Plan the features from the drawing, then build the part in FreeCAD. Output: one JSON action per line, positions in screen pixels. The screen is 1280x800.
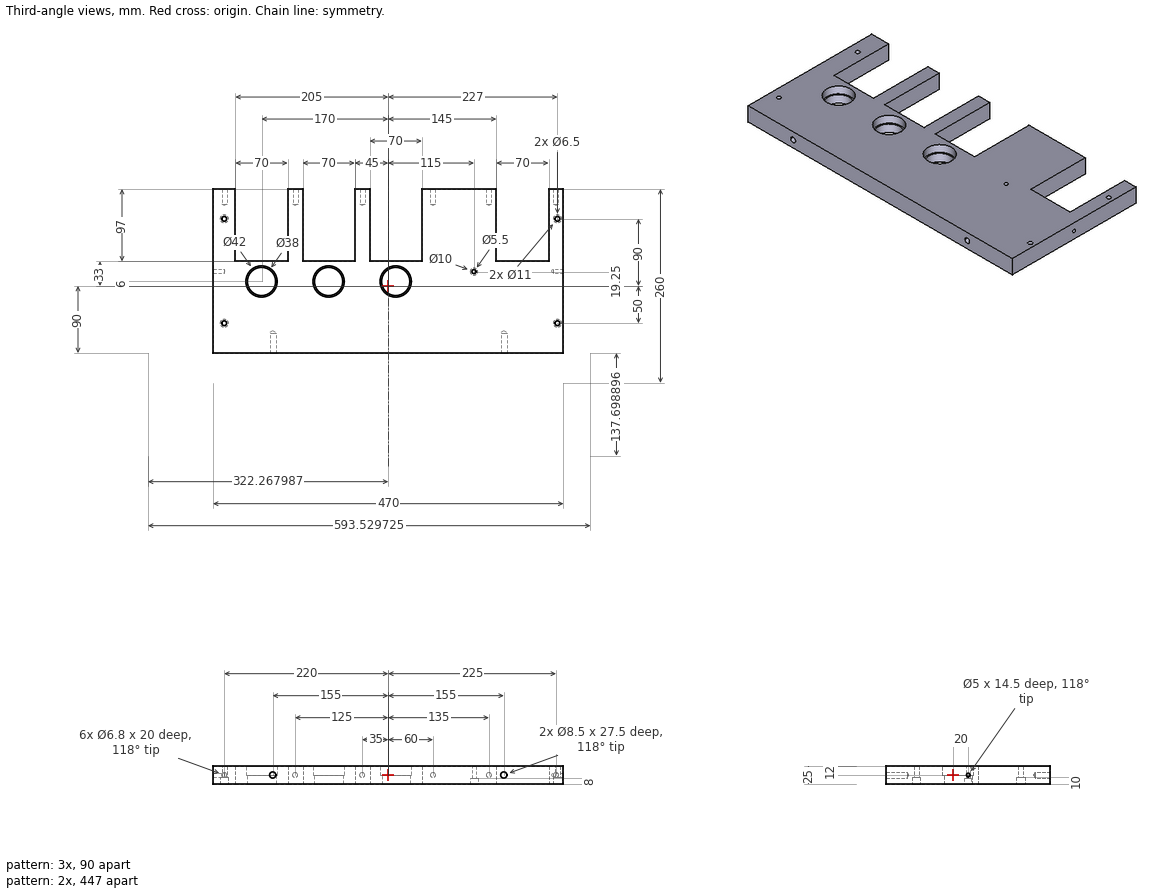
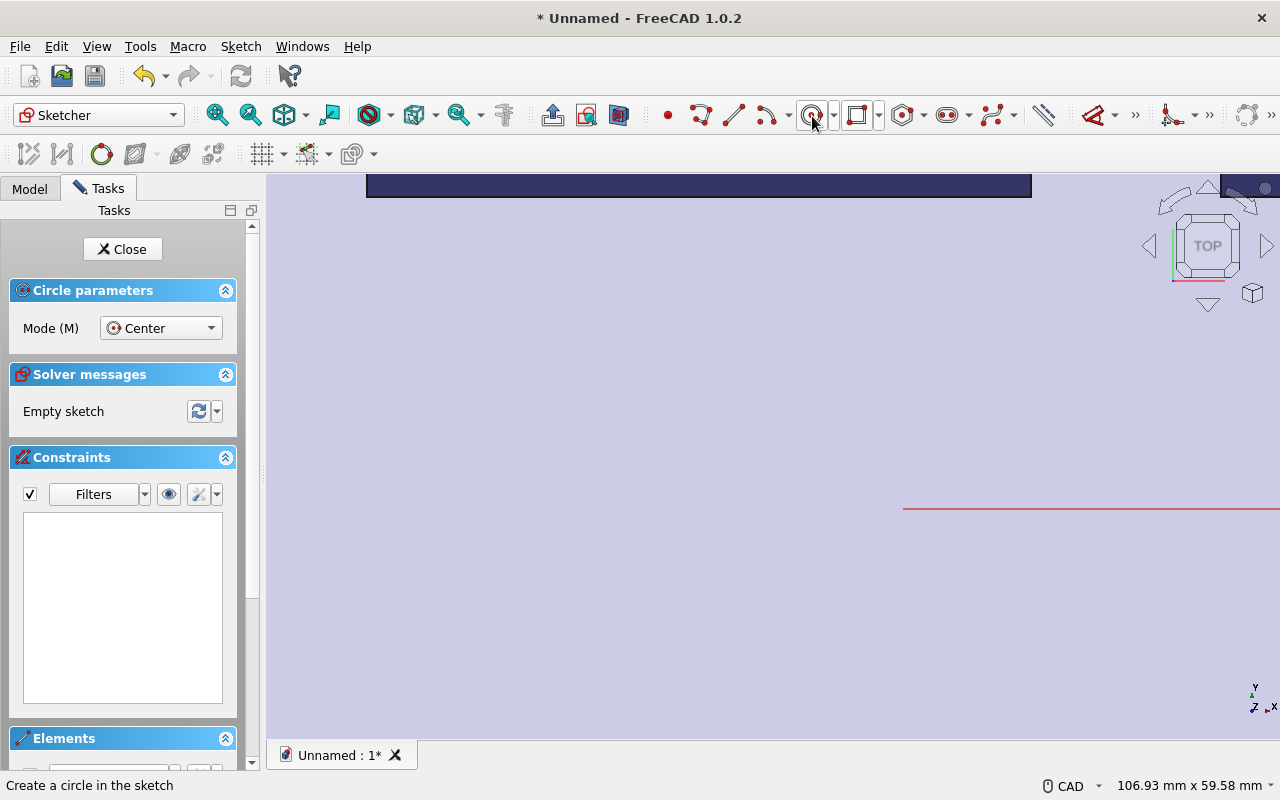
{"action": "left_click", "coordinate": [699, 453]}
{"action": "mouse_move", "coordinate": [827, 325]}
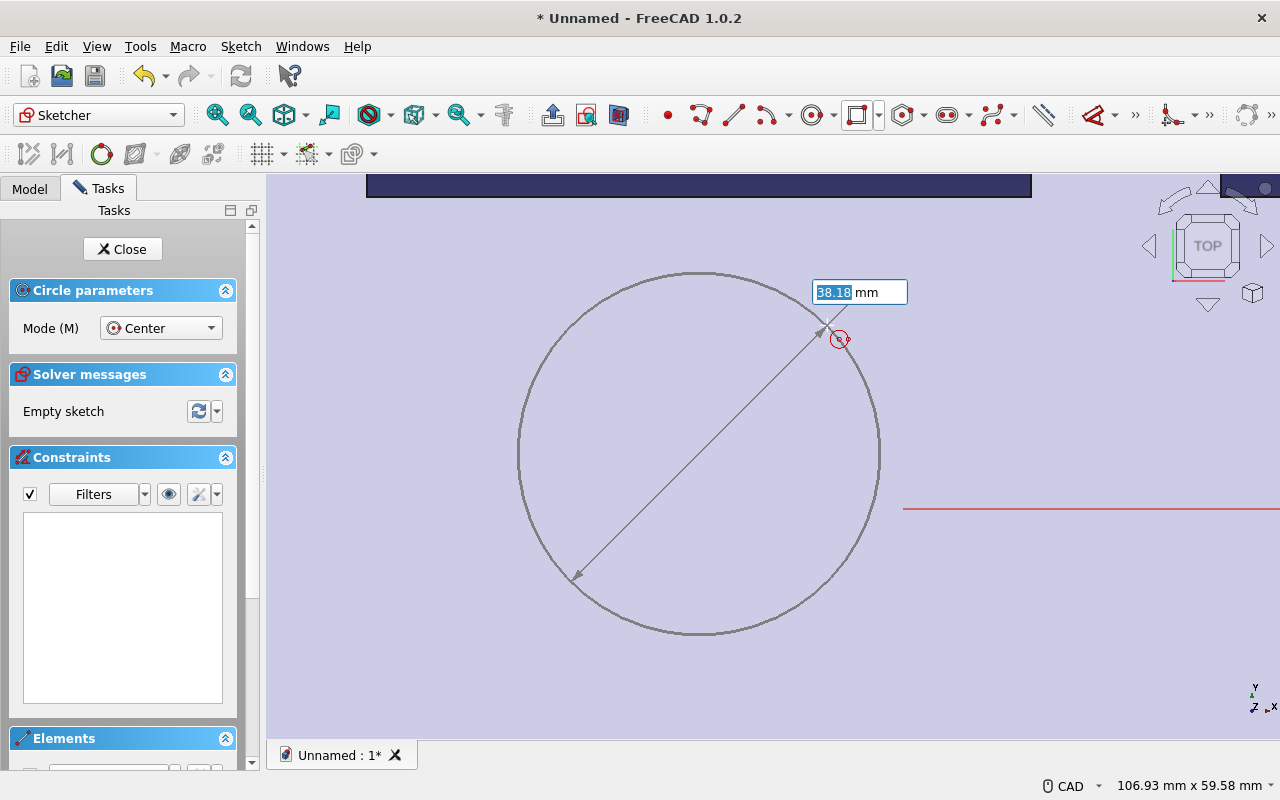
{"action": "type", "text": "38"}
{"action": "key", "text": "Return"}
{"action": "key", "text": "Escape"}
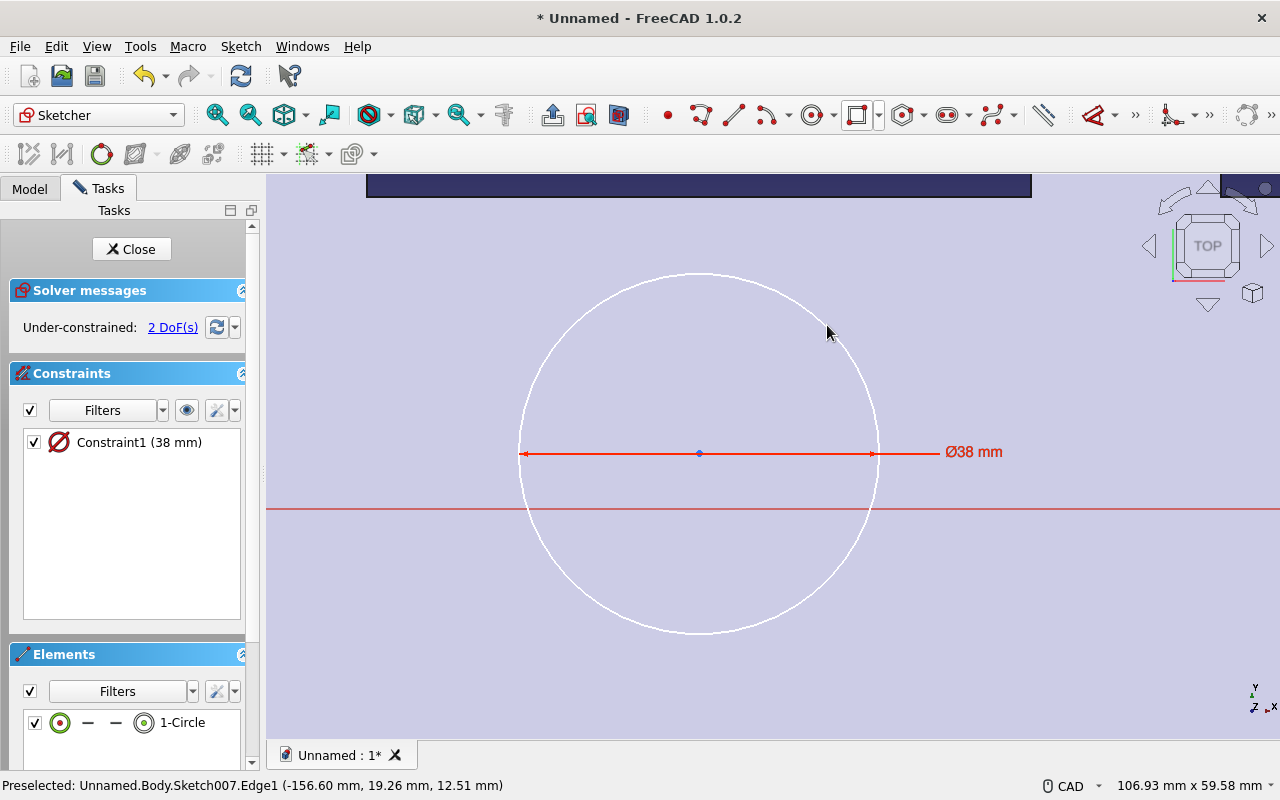
{"action": "left_click", "coordinate": [1092, 116]}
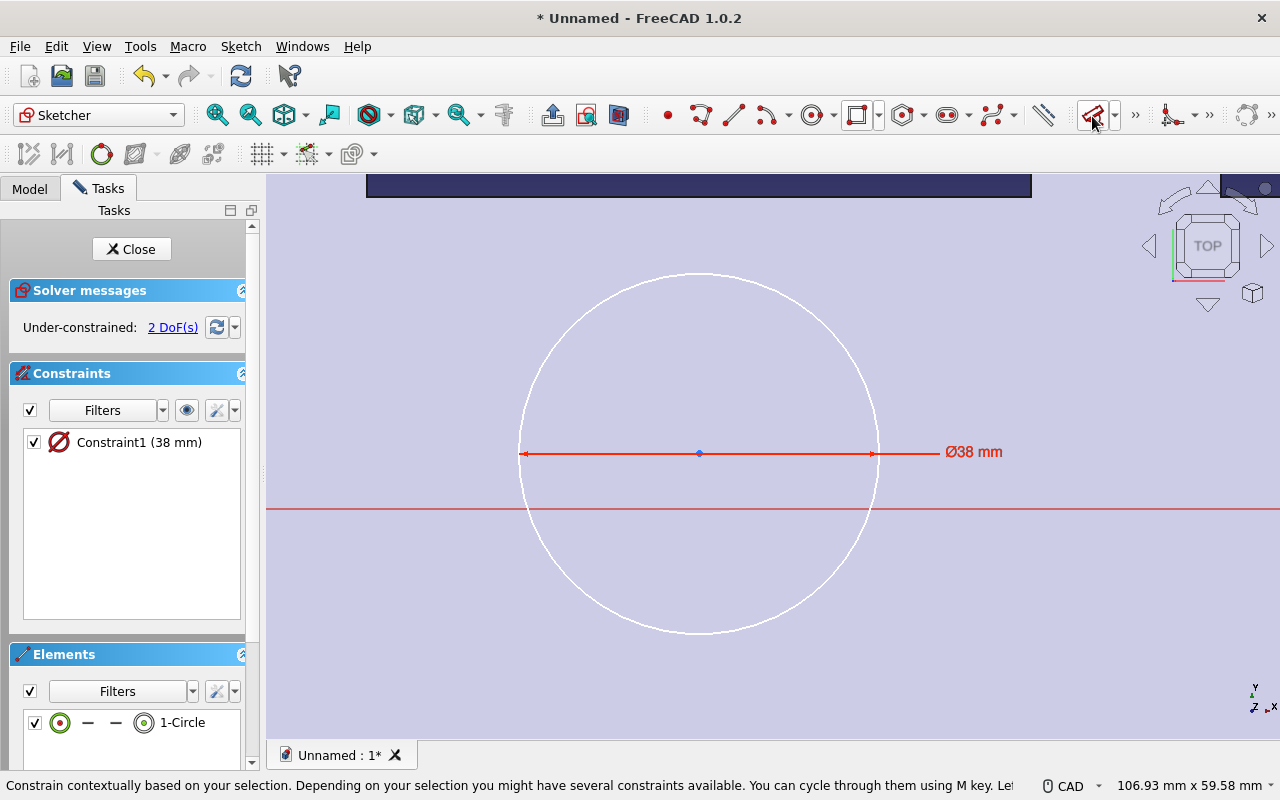
{"action": "left_click", "coordinate": [699, 454]}
{"action": "left_click", "coordinate": [665, 482]}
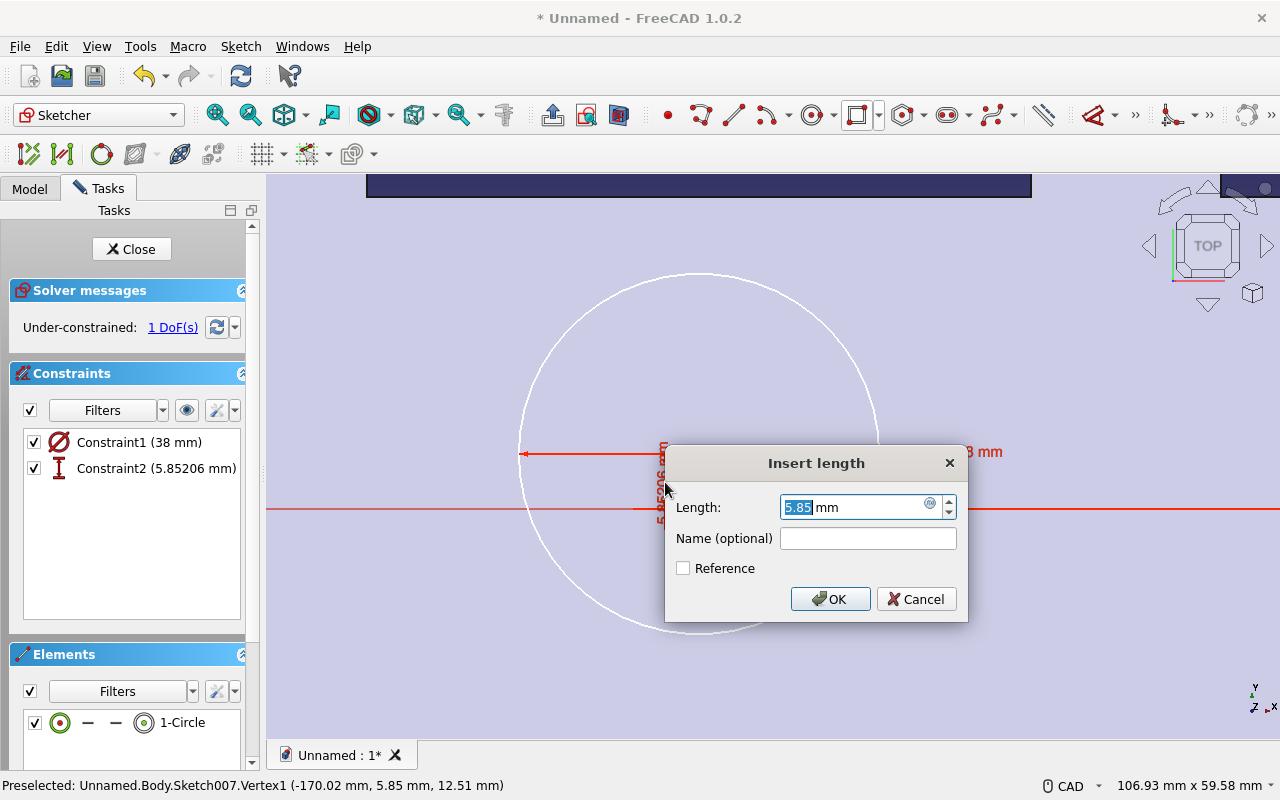
{"action": "type", "text": "6"}
{"action": "key", "text": "Return"}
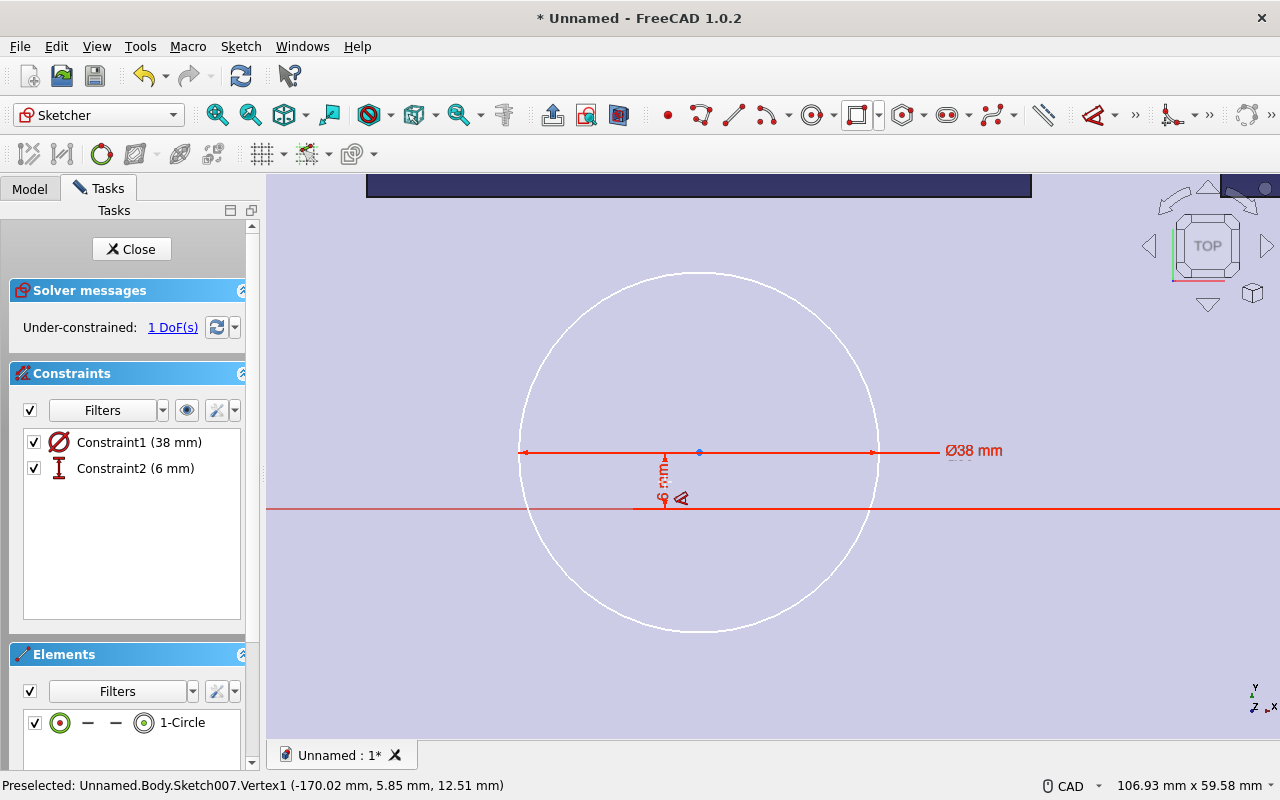
{"action": "left_click", "coordinate": [699, 453]}
{"action": "left_click", "coordinate": [907, 543]}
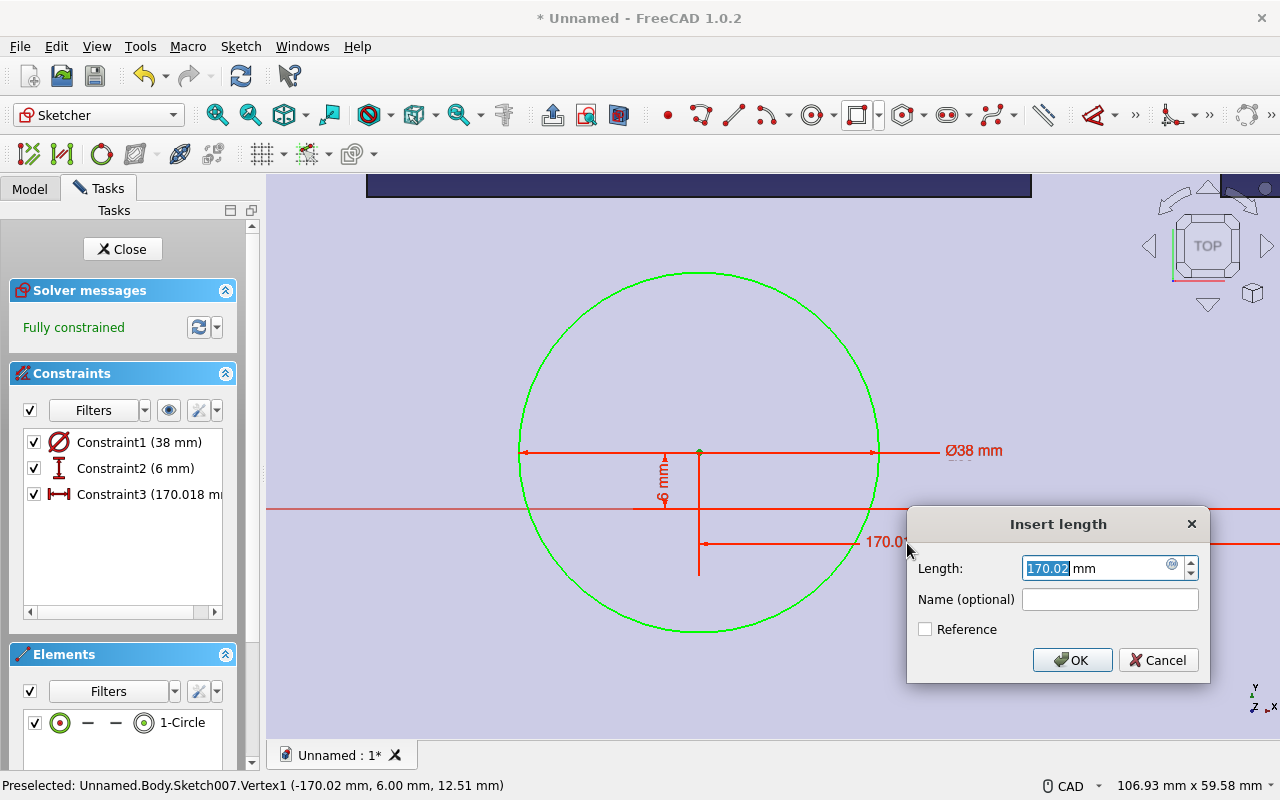
{"action": "type", "text": "170"}
{"action": "key", "text": "Return"}
{"action": "key", "text": "Escape"}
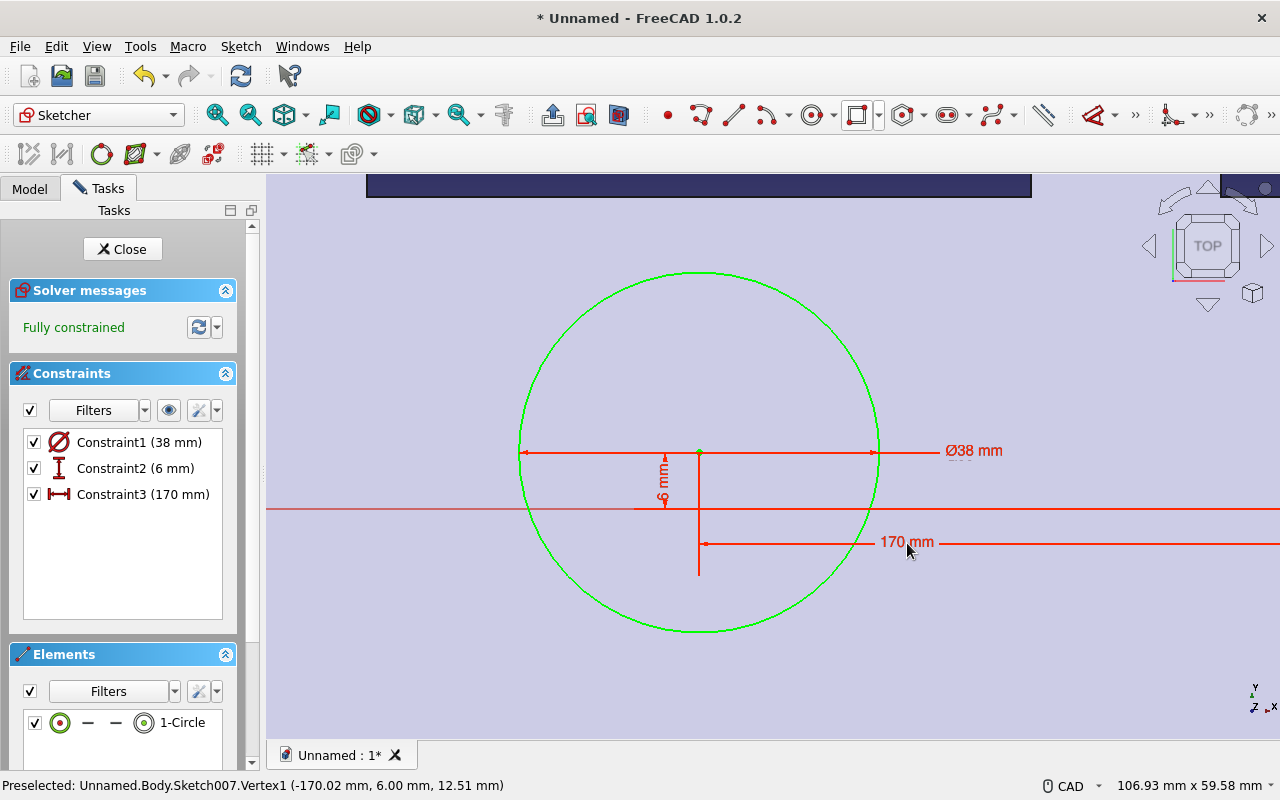
{"action": "left_click", "coordinate": [123, 249]}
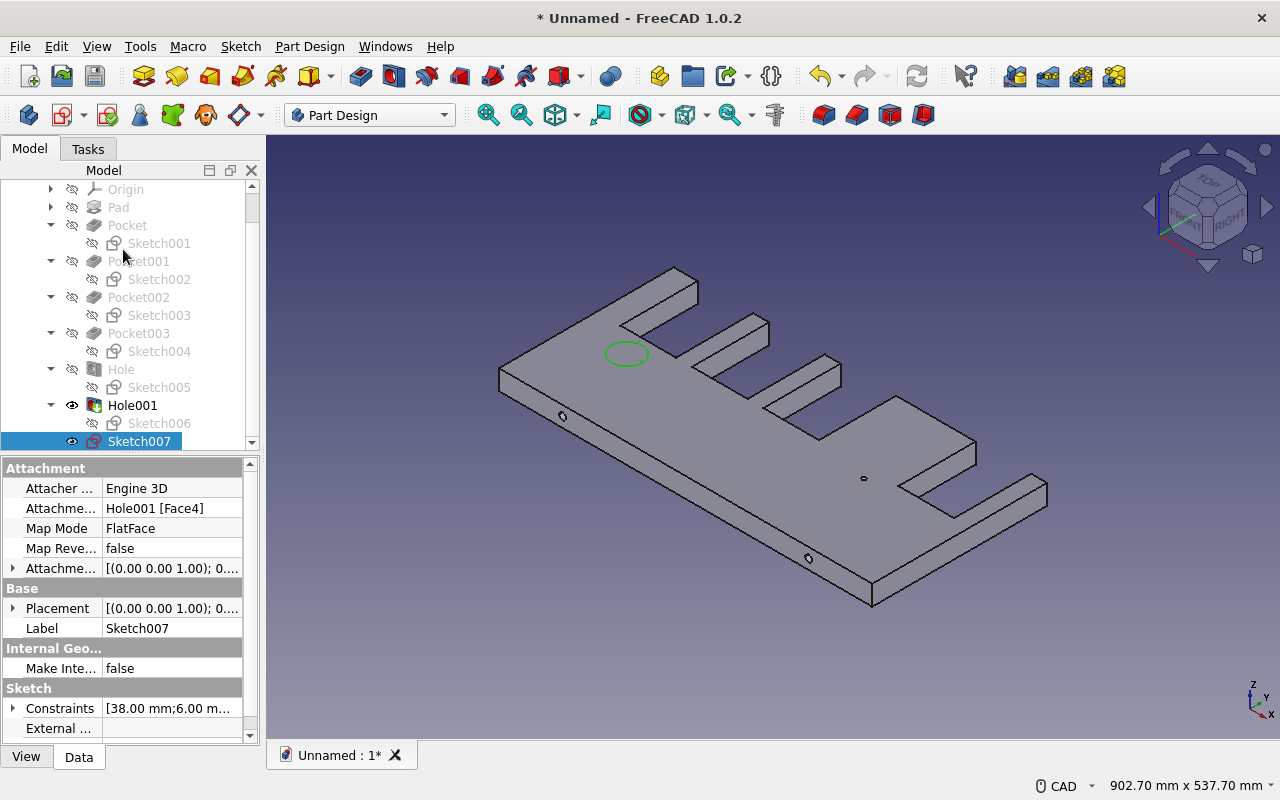
{"action": "left_click", "coordinate": [361, 76]}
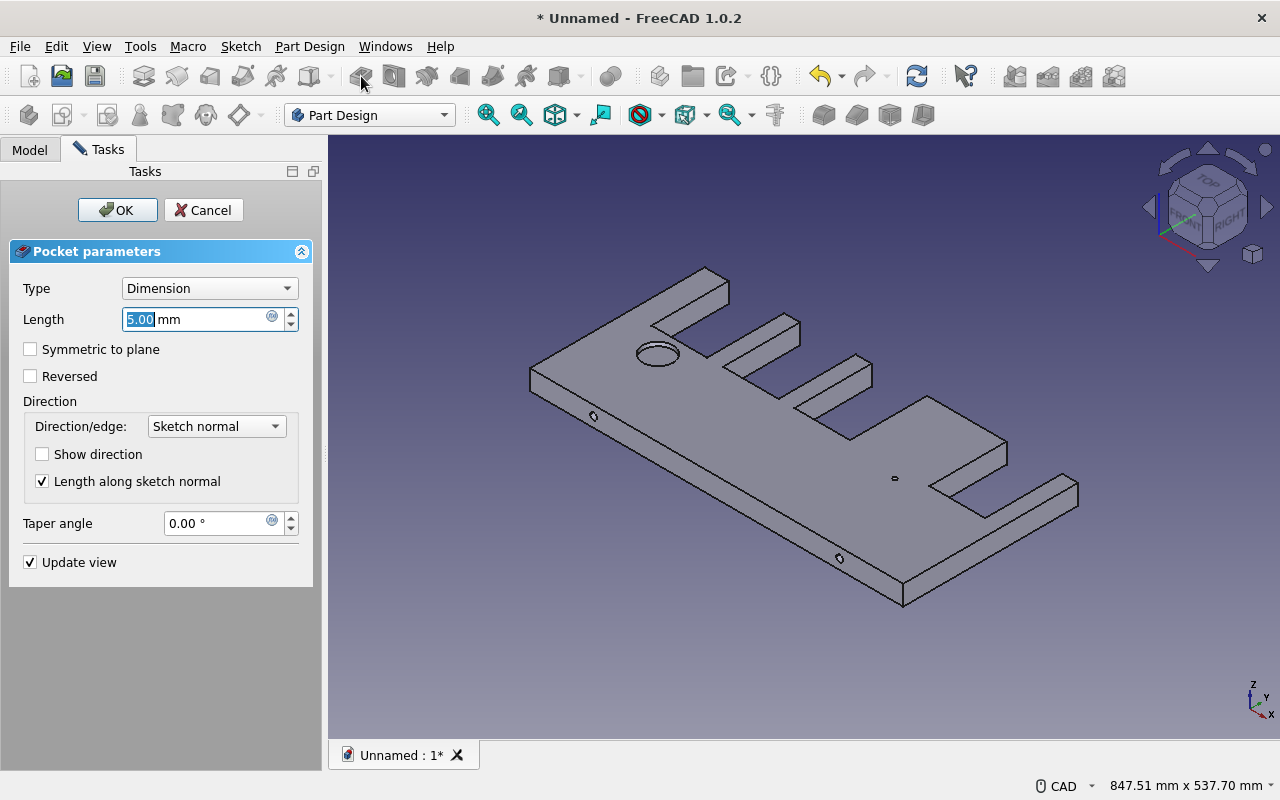
{"action": "left_click", "coordinate": [210, 288]}